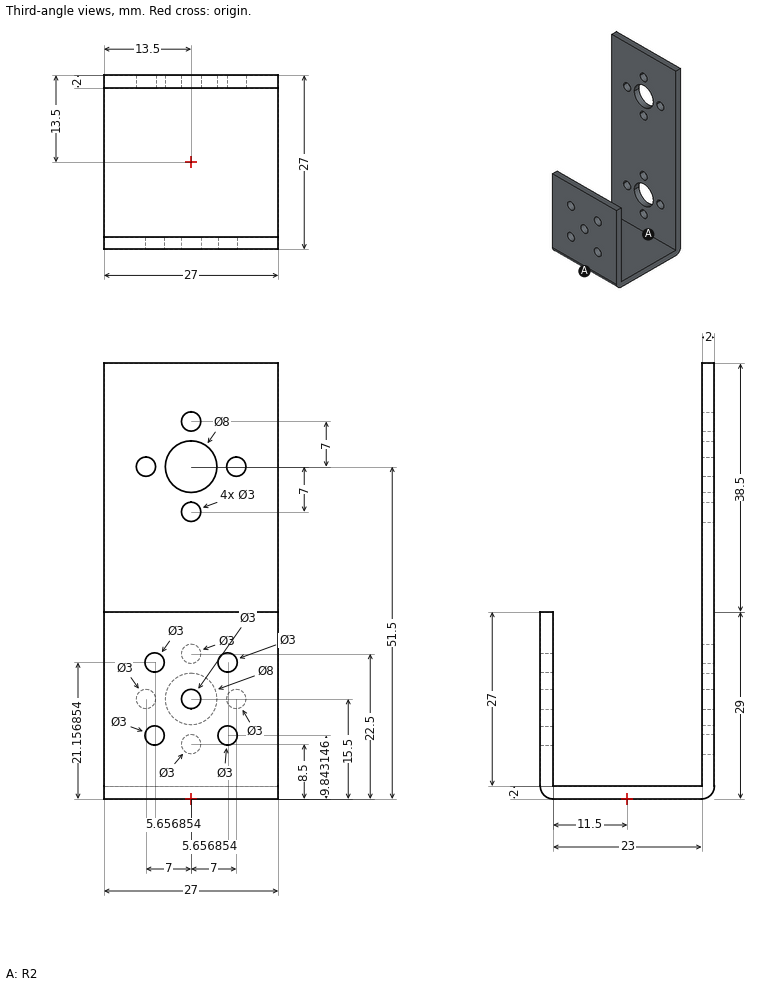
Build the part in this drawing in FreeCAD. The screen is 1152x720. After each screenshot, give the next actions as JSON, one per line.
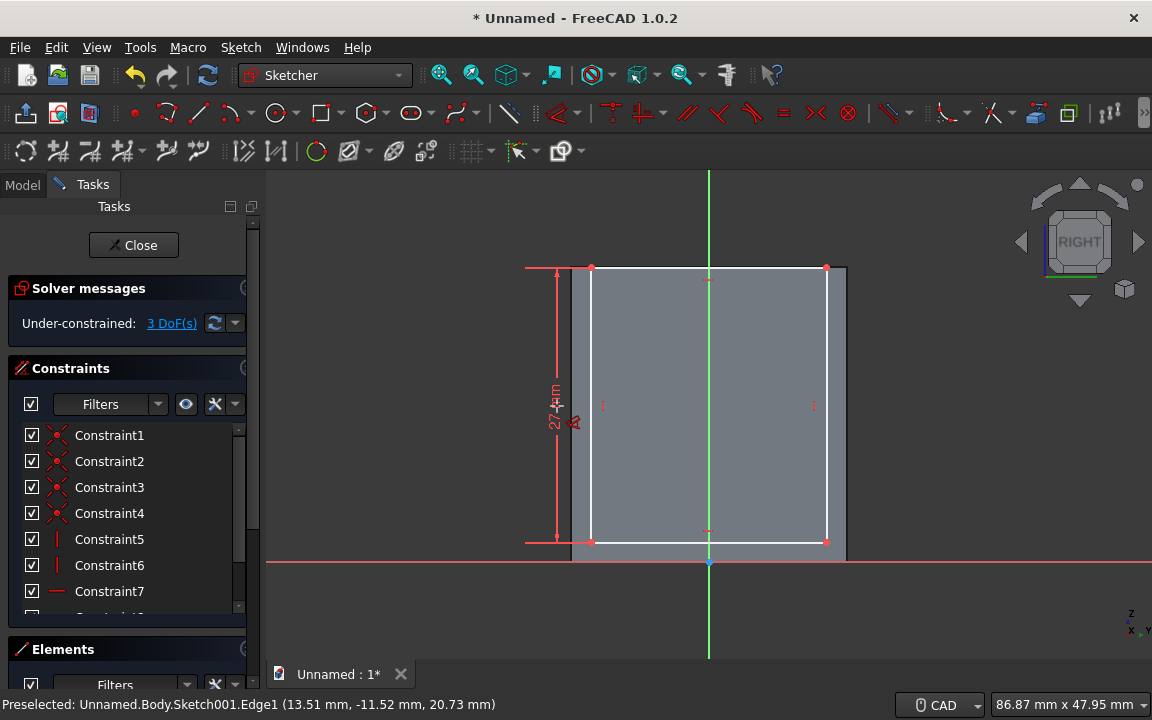
{"action": "left_click", "coordinate": [662, 543]}
{"action": "left_click", "coordinate": [655, 577]}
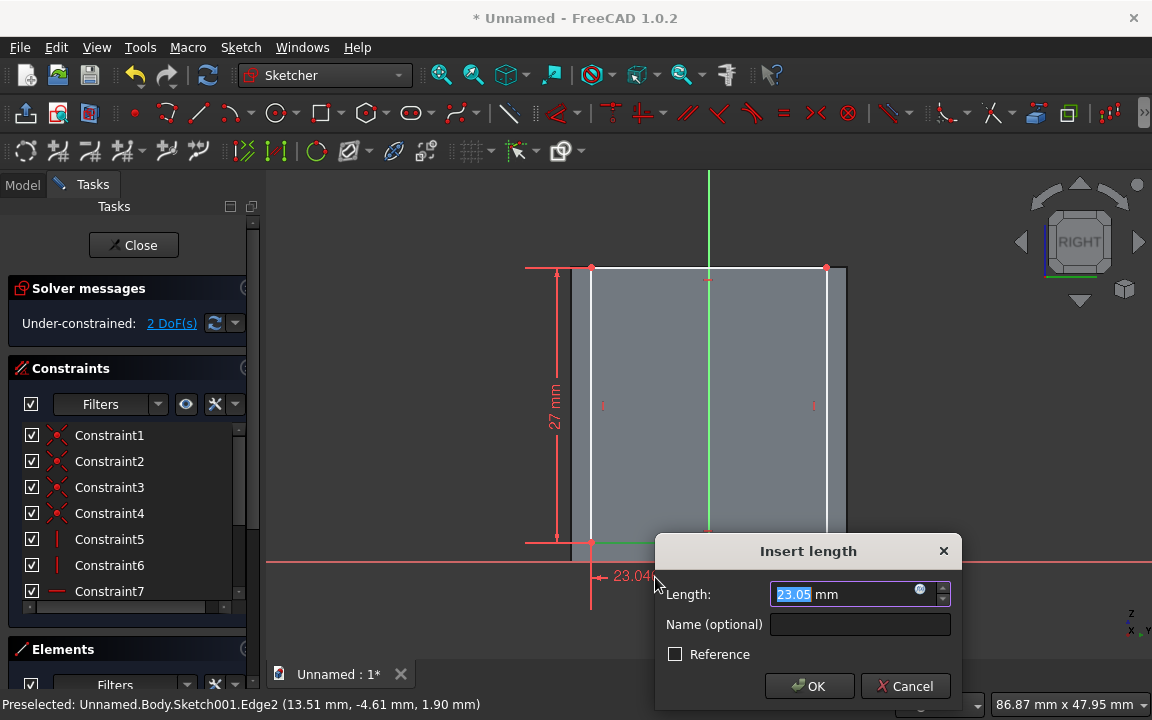
{"action": "type", "text": "23"}
{"action": "key", "text": "Return"}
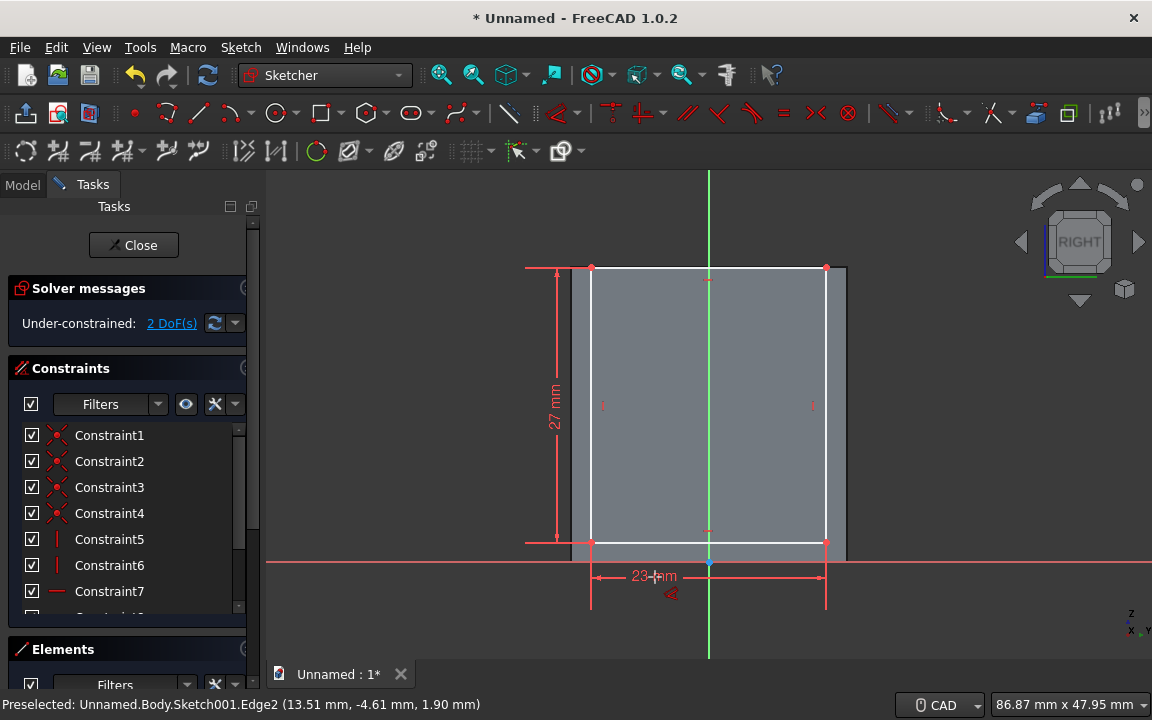
{"action": "scroll", "coordinate": [591, 543], "scroll_direction": "up", "scroll_amount": 4}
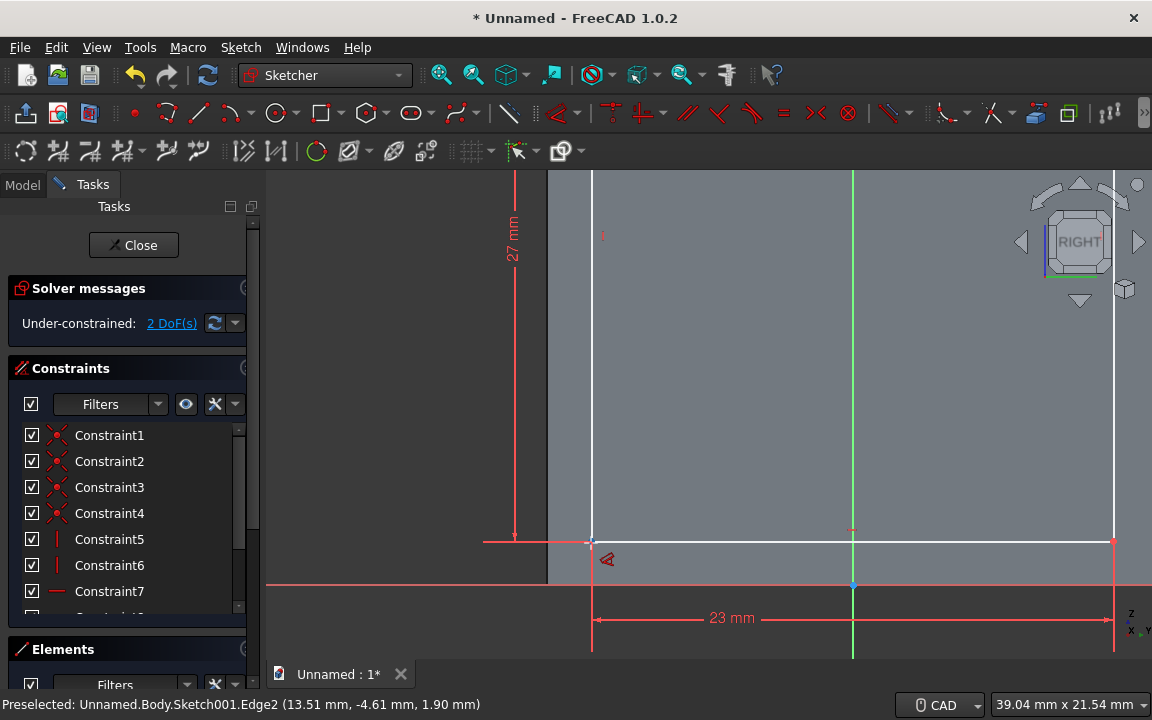
{"action": "left_click", "coordinate": [592, 542]}
{"action": "left_click", "coordinate": [558, 564]}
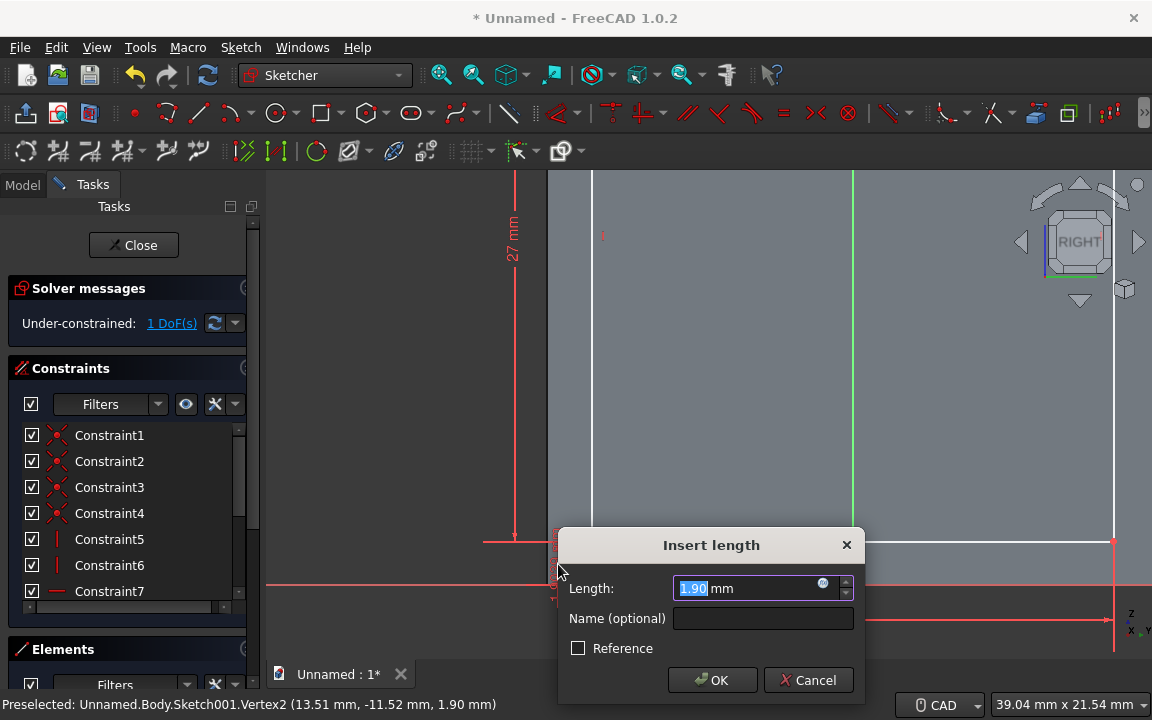
{"action": "type", "text": "2"}
{"action": "key", "text": "Return"}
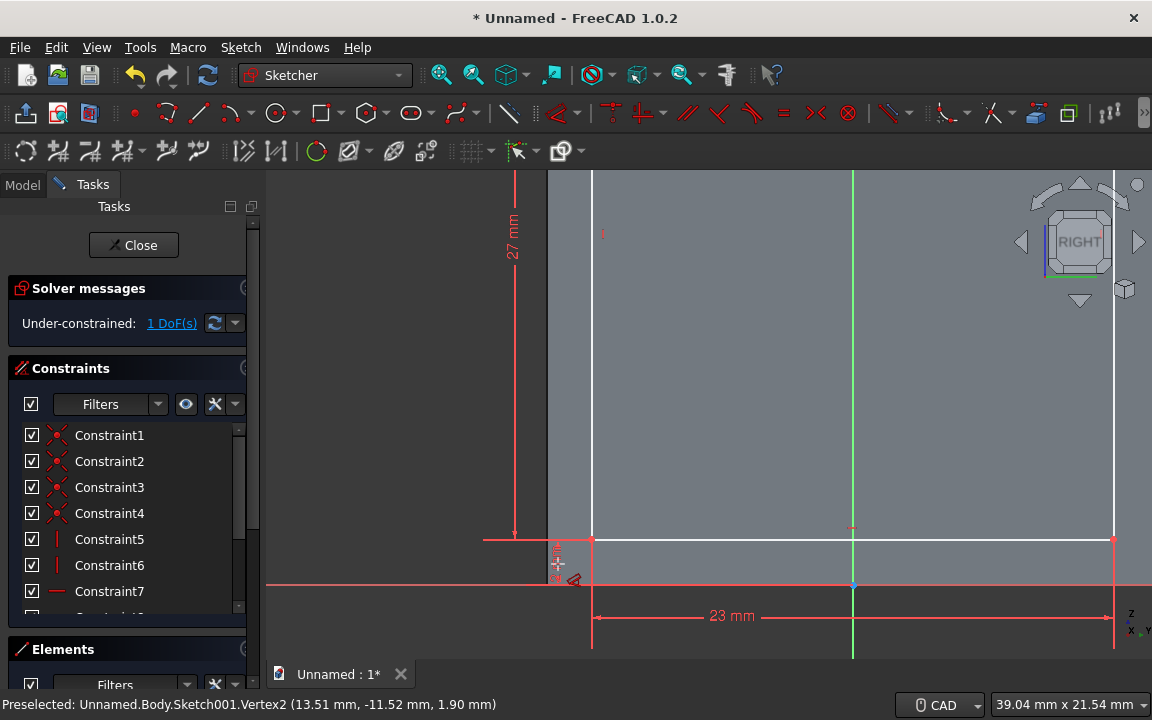
{"action": "scroll", "coordinate": [467, 544], "scroll_direction": "down", "scroll_amount": 4}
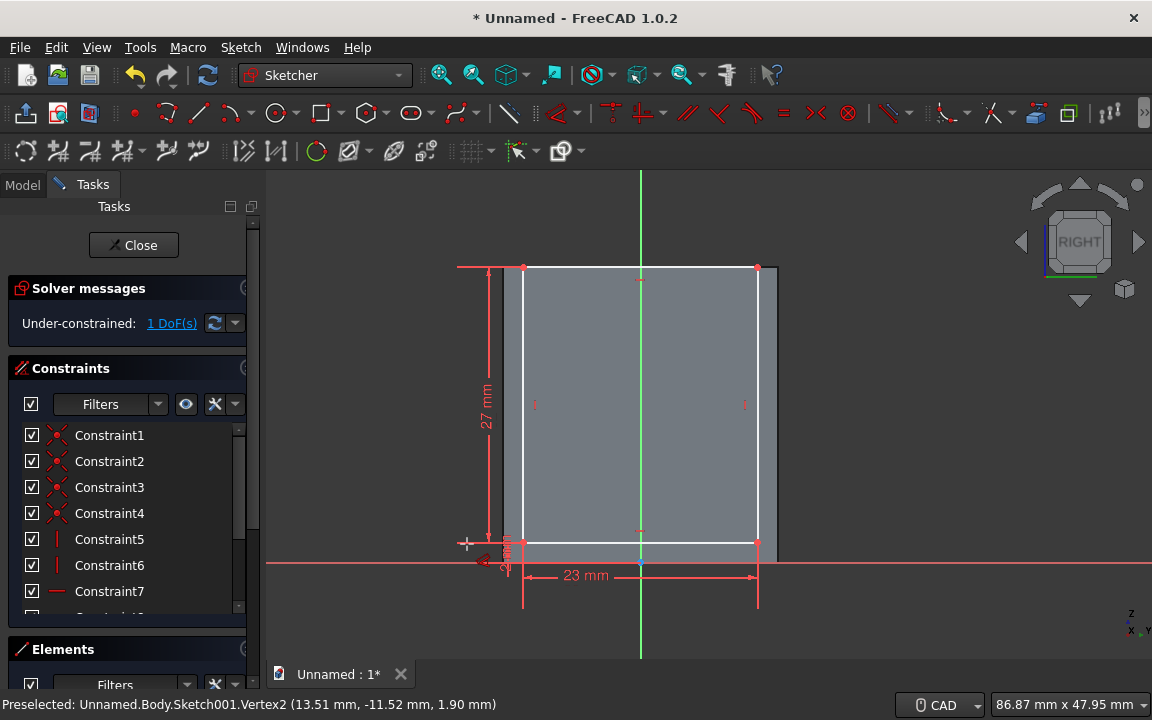
{"action": "left_click", "coordinate": [523, 267]}
{"action": "left_click", "coordinate": [582, 233]}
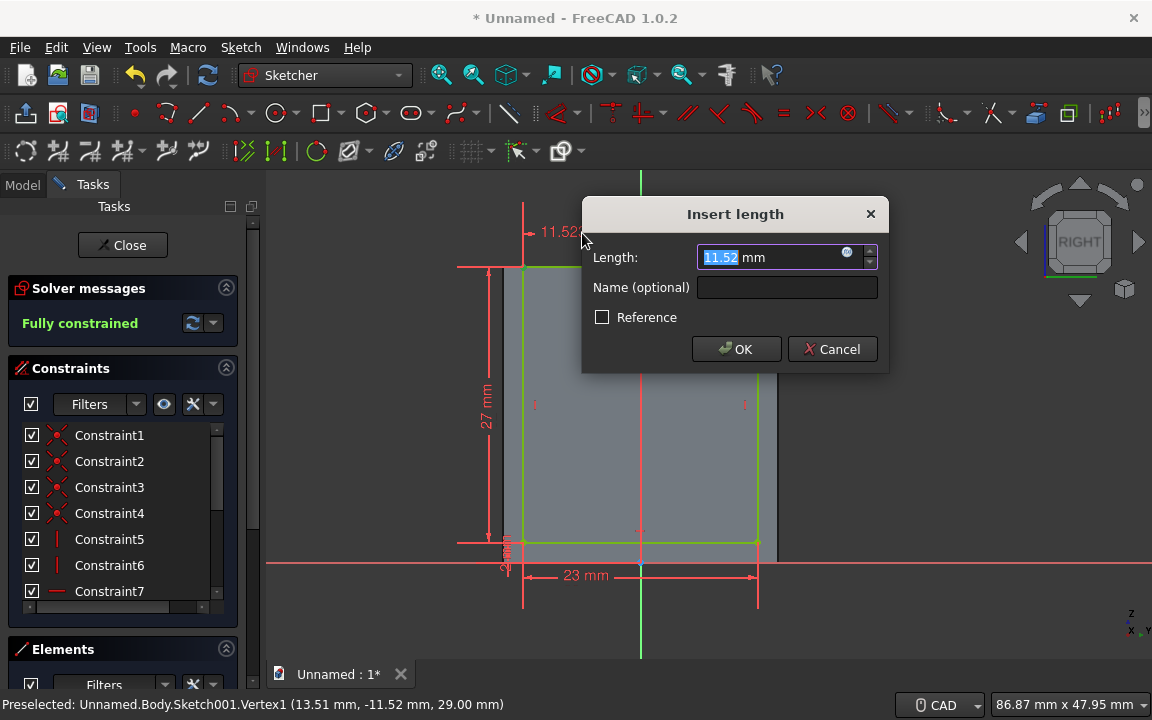
{"action": "type", "text": "11.5"}
{"action": "key", "text": "Return"}
{"action": "key", "text": "Escape"}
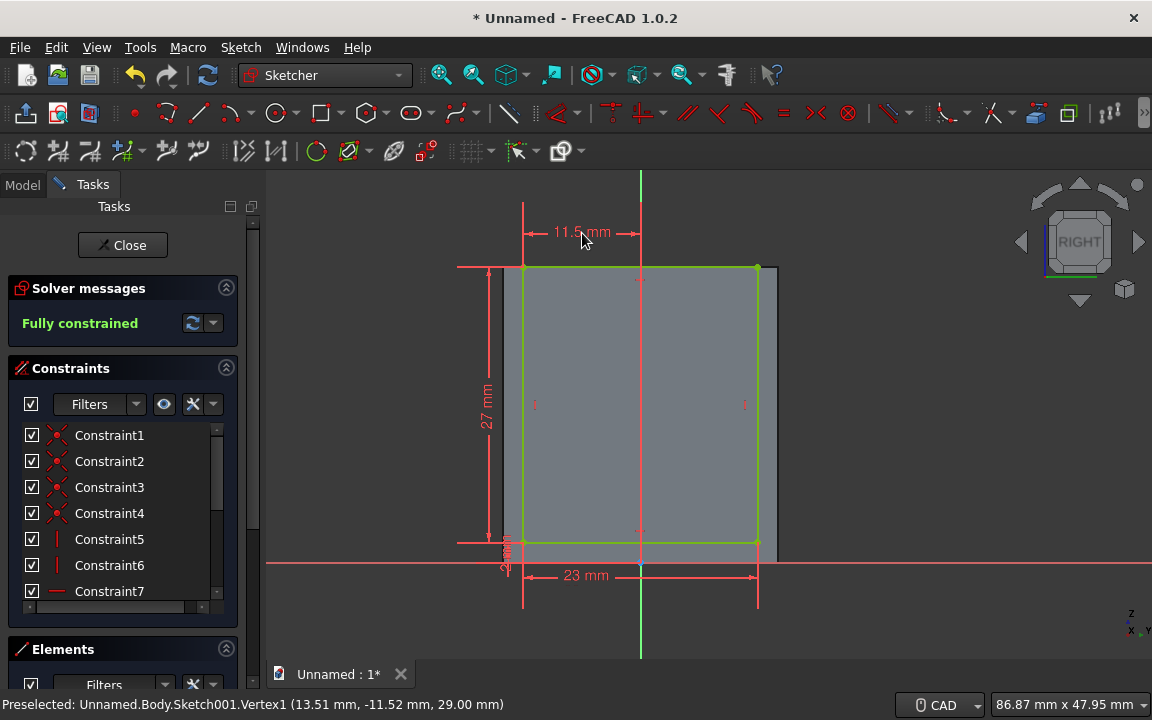
{"action": "left_click", "coordinate": [123, 245]}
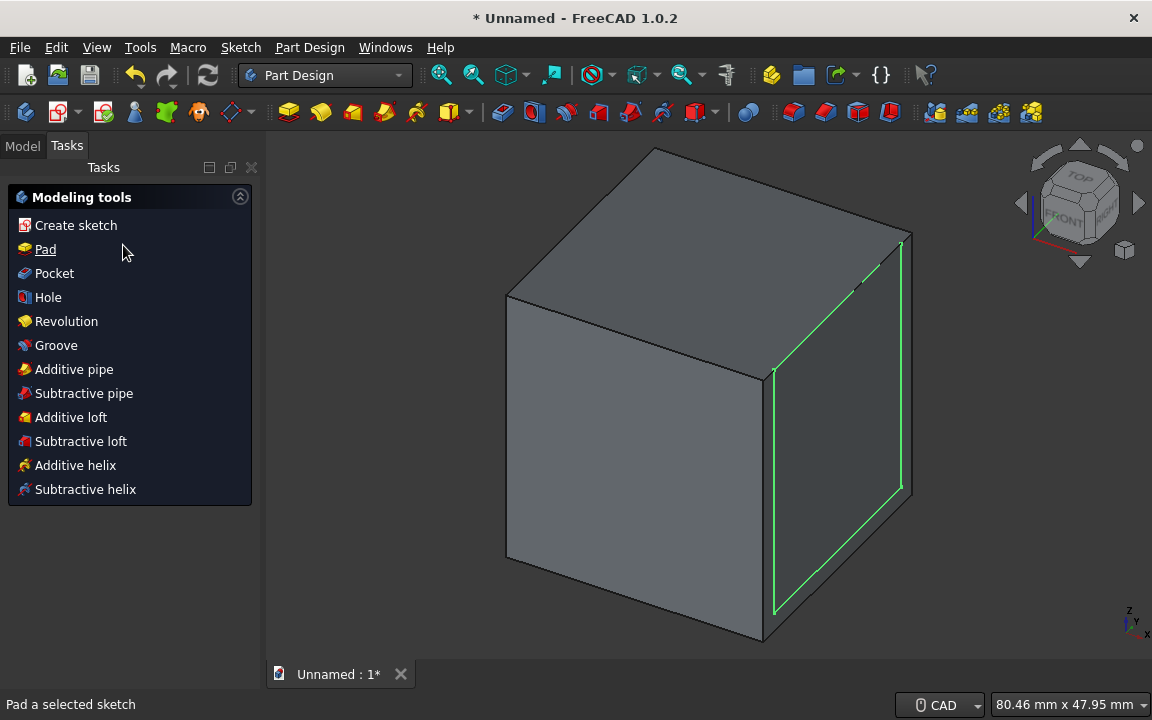
{"action": "left_click", "coordinate": [504, 112]}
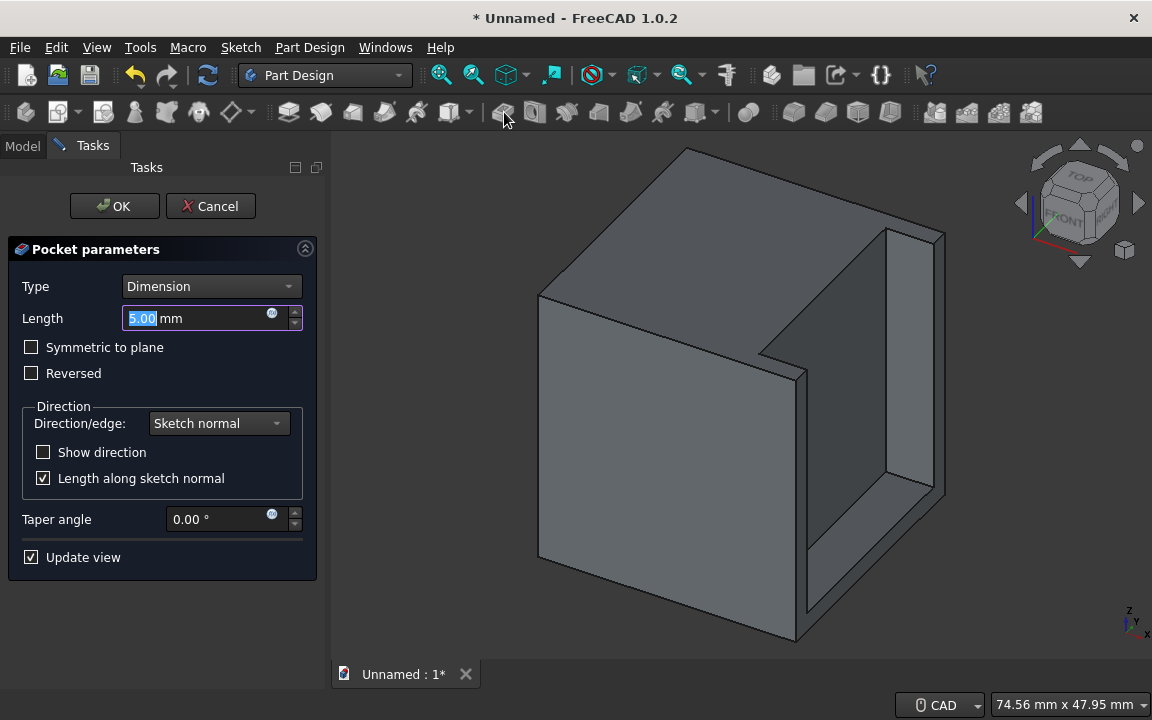
{"action": "type", "text": "27"}
{"action": "key", "text": "Tab"}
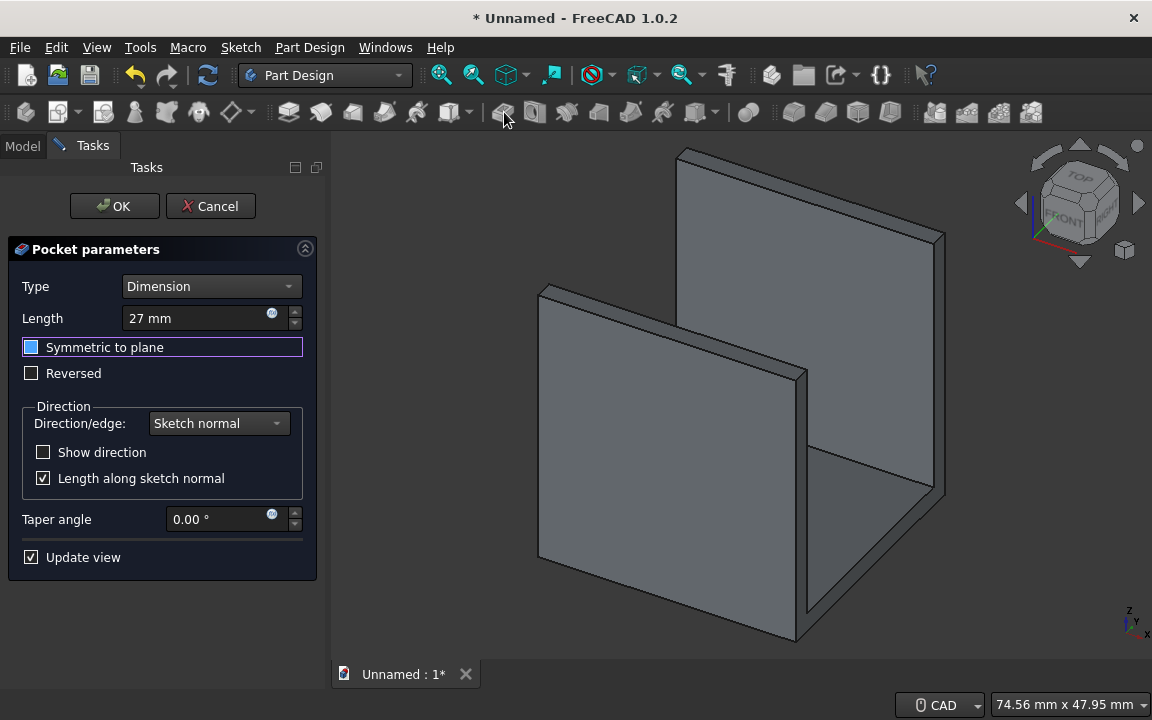
{"action": "left_click", "coordinate": [115, 206]}